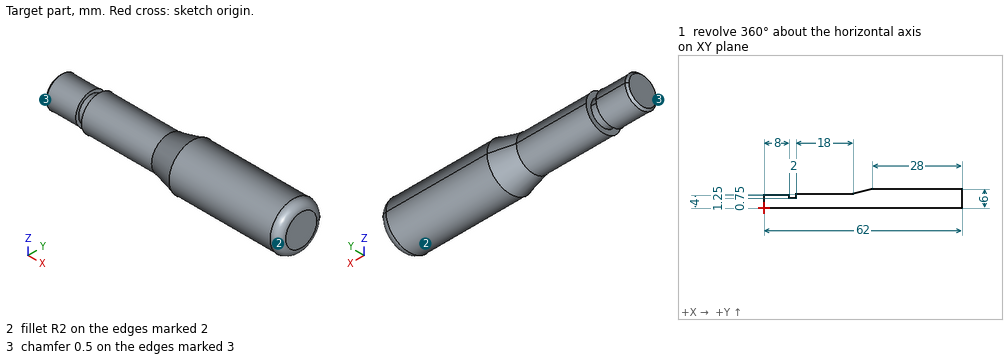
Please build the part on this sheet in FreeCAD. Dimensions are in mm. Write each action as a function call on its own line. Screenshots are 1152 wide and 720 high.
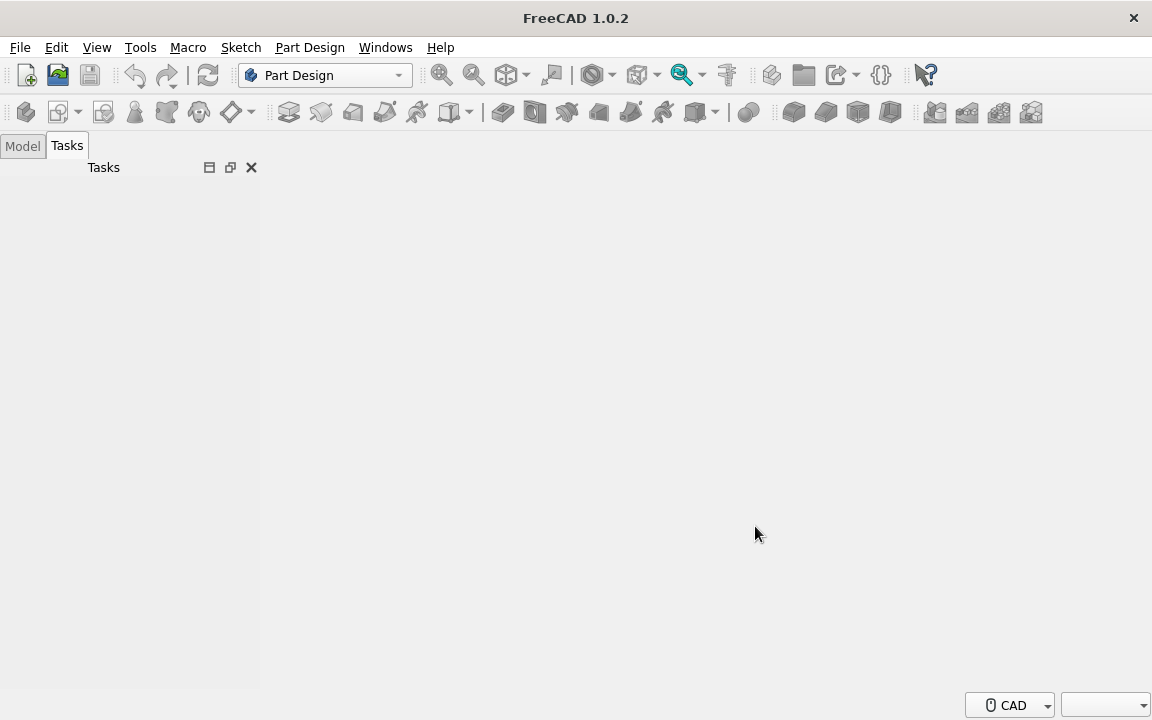
click(26, 76)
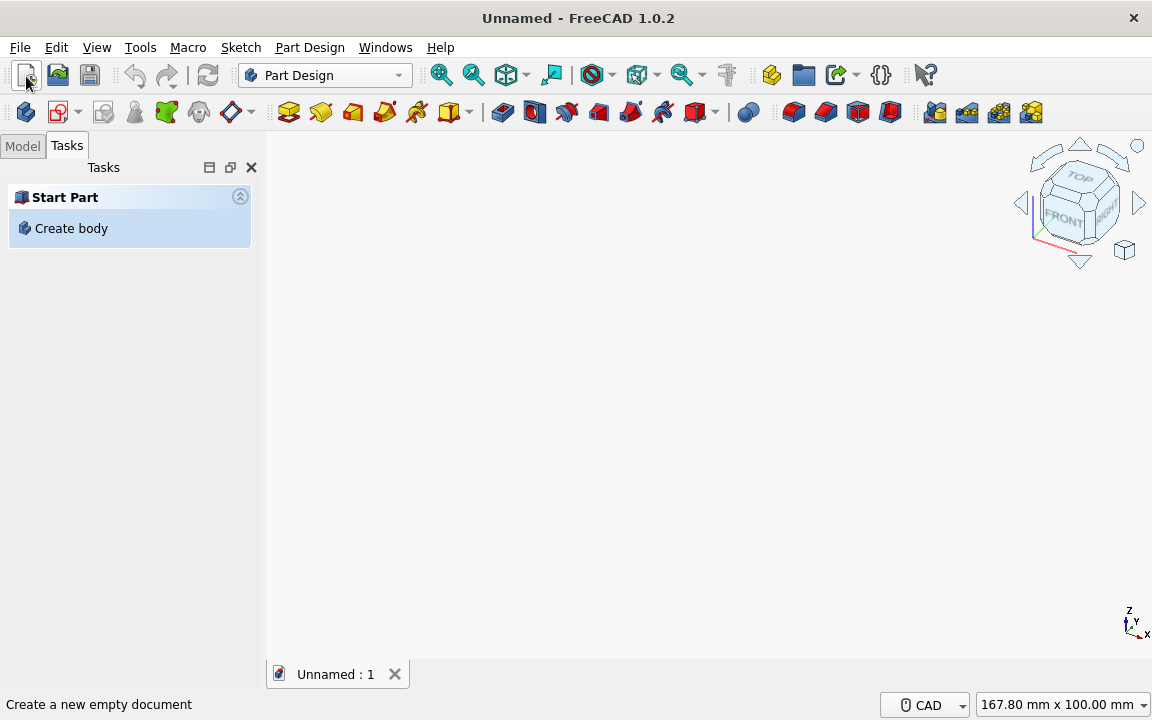
click(58, 112)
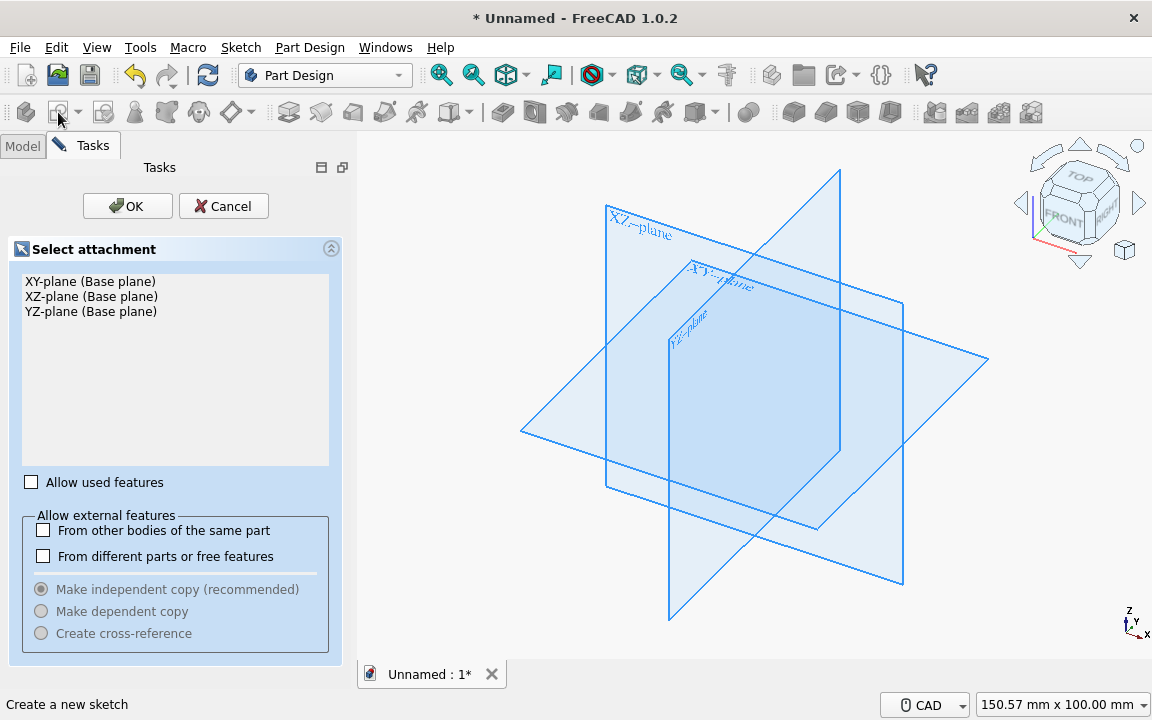
click(82, 282)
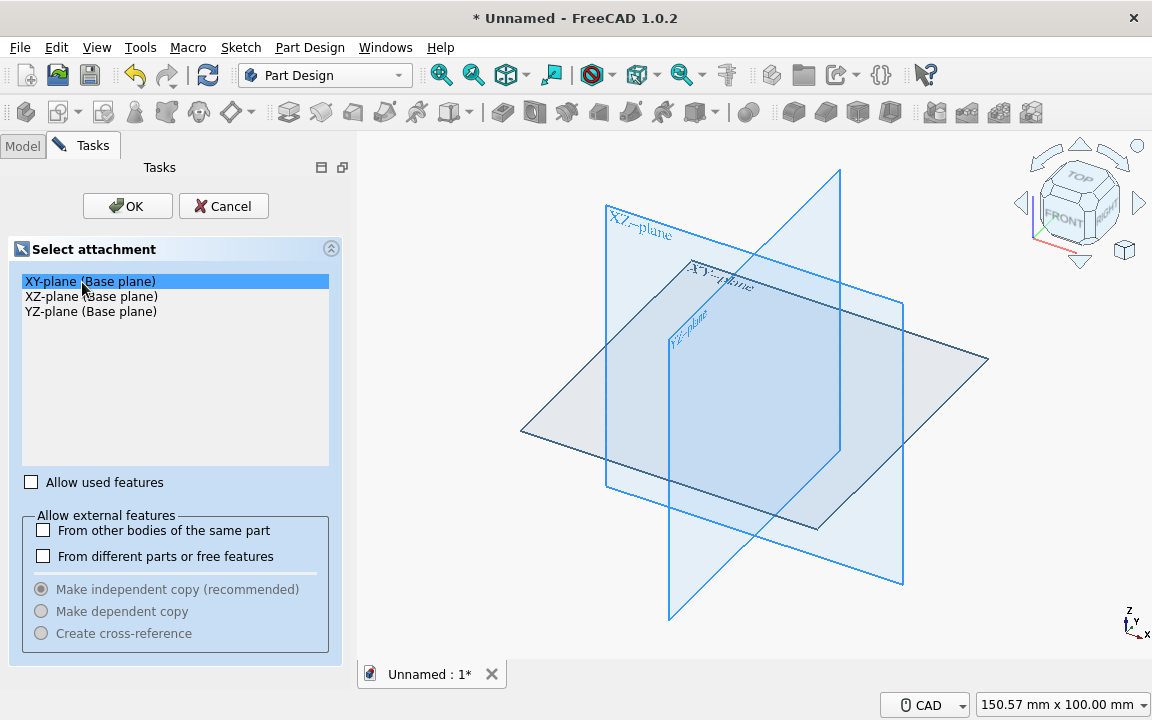
click(128, 206)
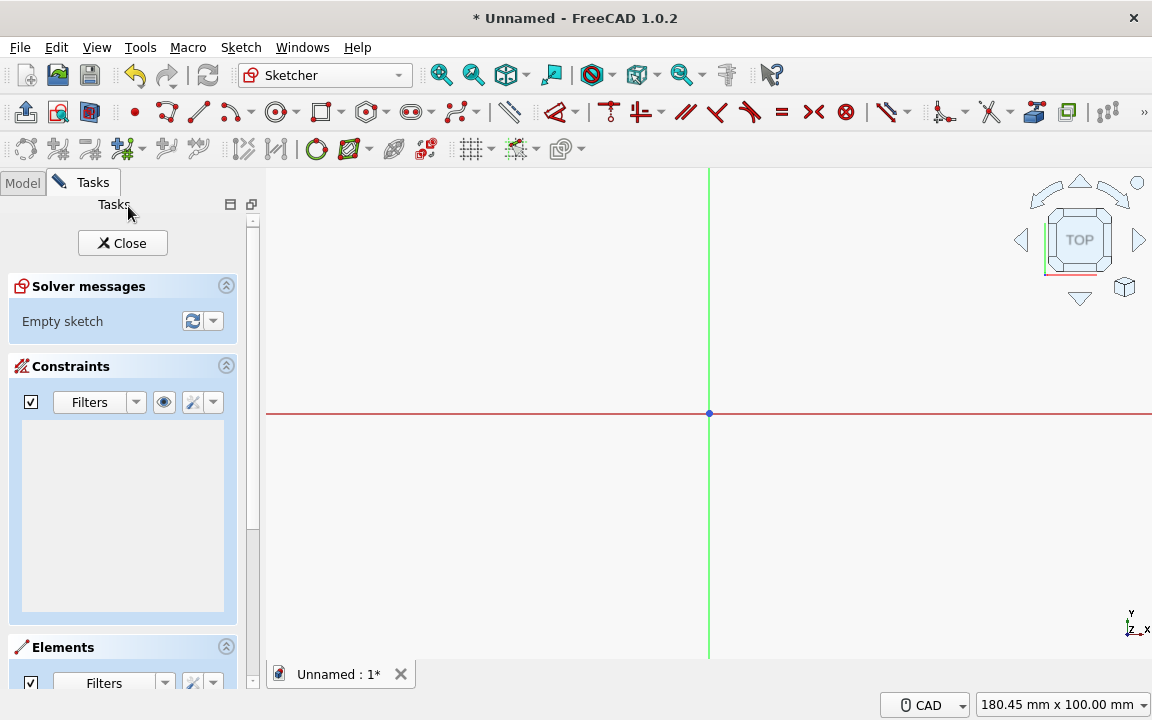
scroll(294, 480, down, 1)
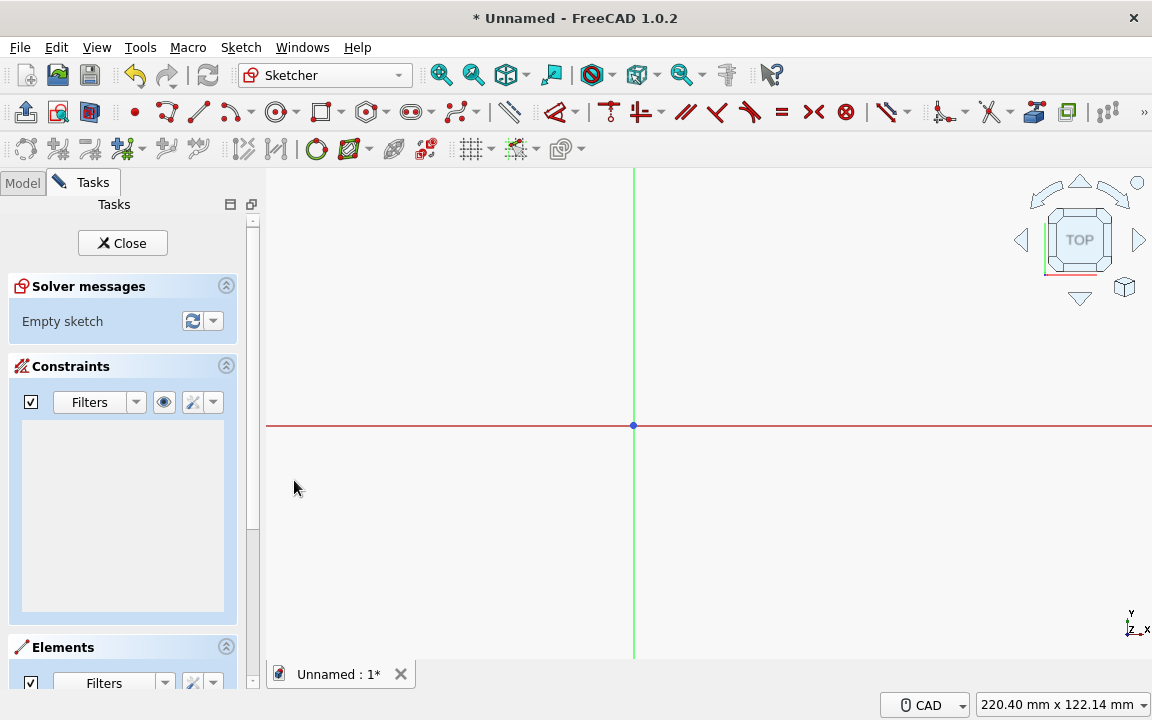
scroll(902, 414, up, 3)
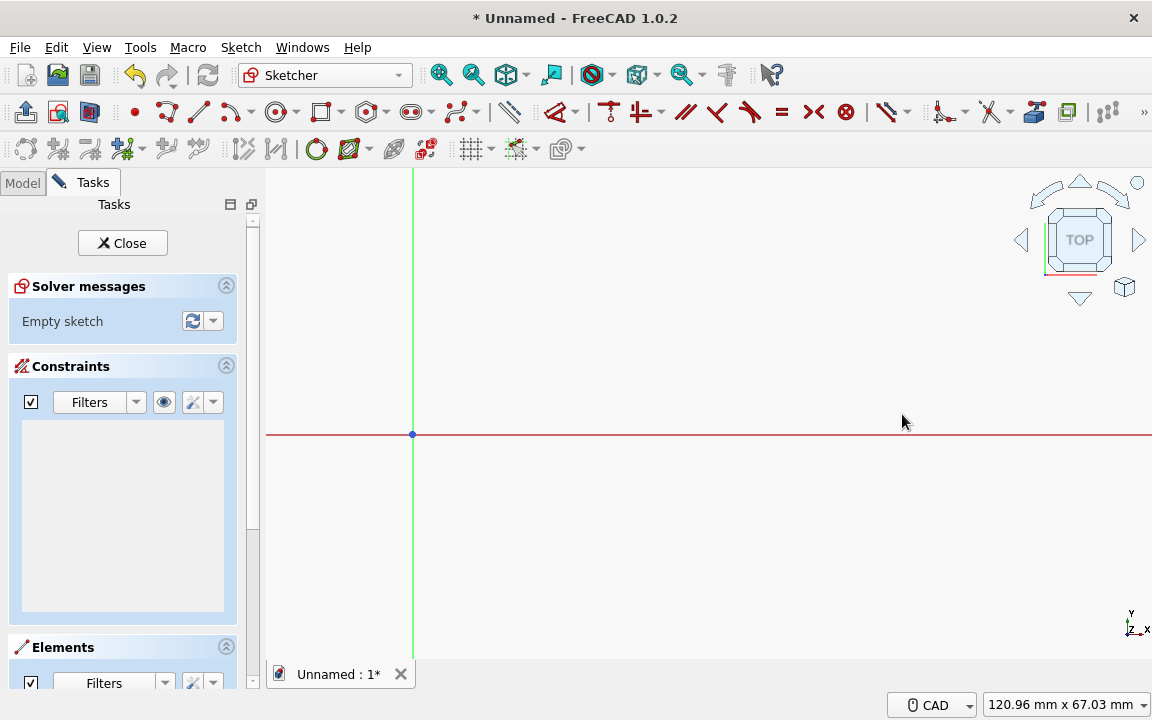
click(168, 112)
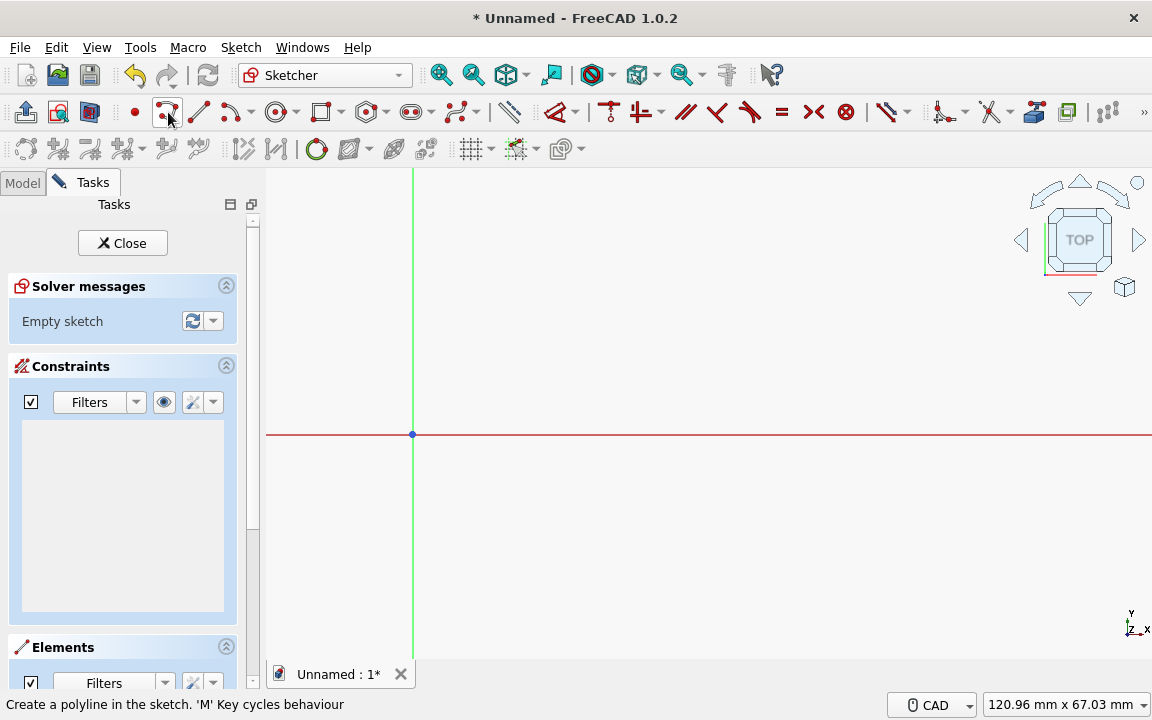
click(413, 435)
click(867, 426)
click(867, 391)
click(662, 391)
click(618, 402)
click(486, 402)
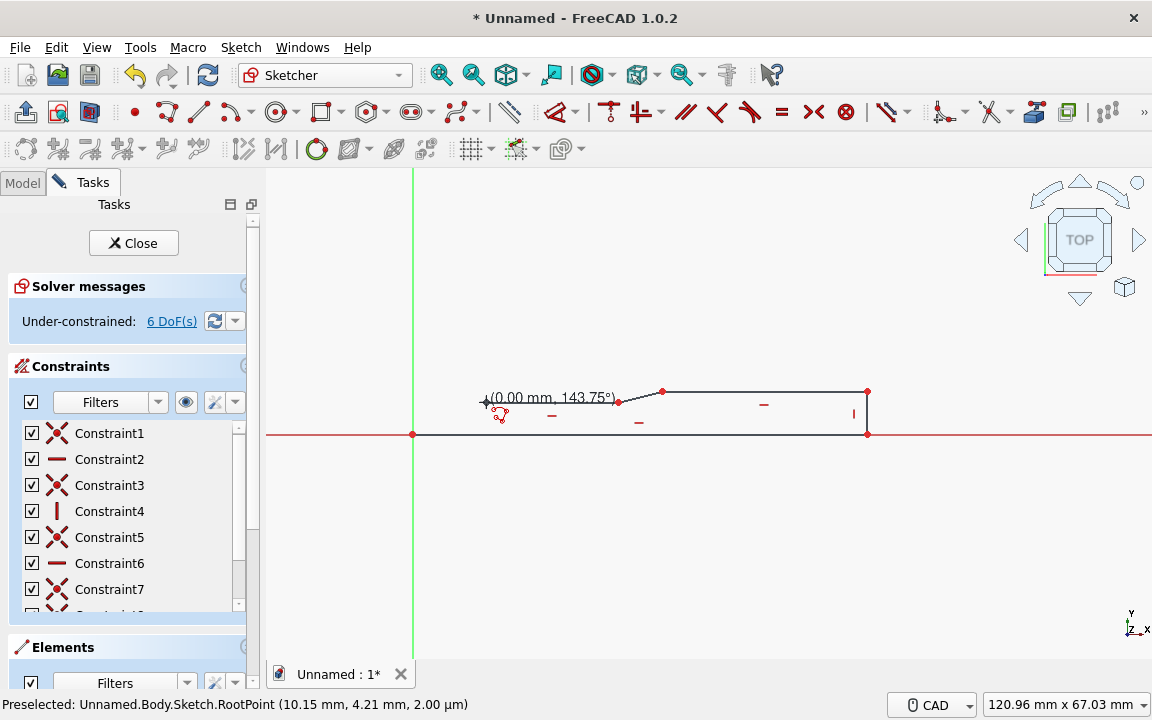
scroll(486, 411, up, 3)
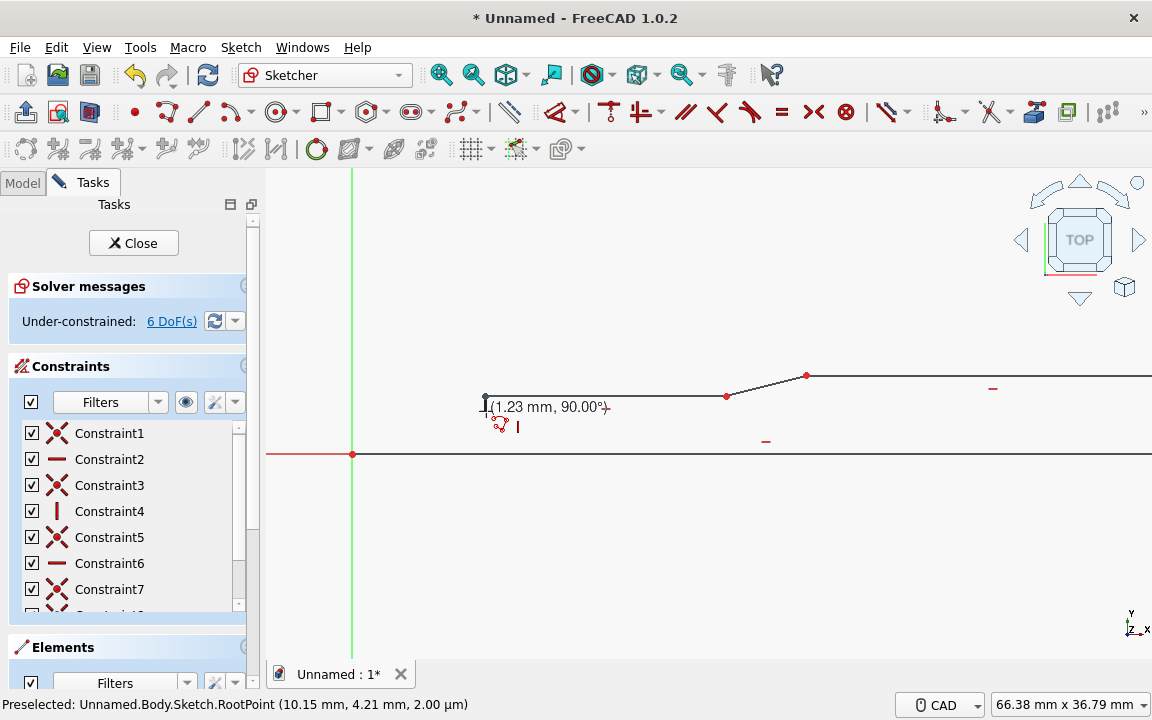
click(486, 411)
click(459, 411)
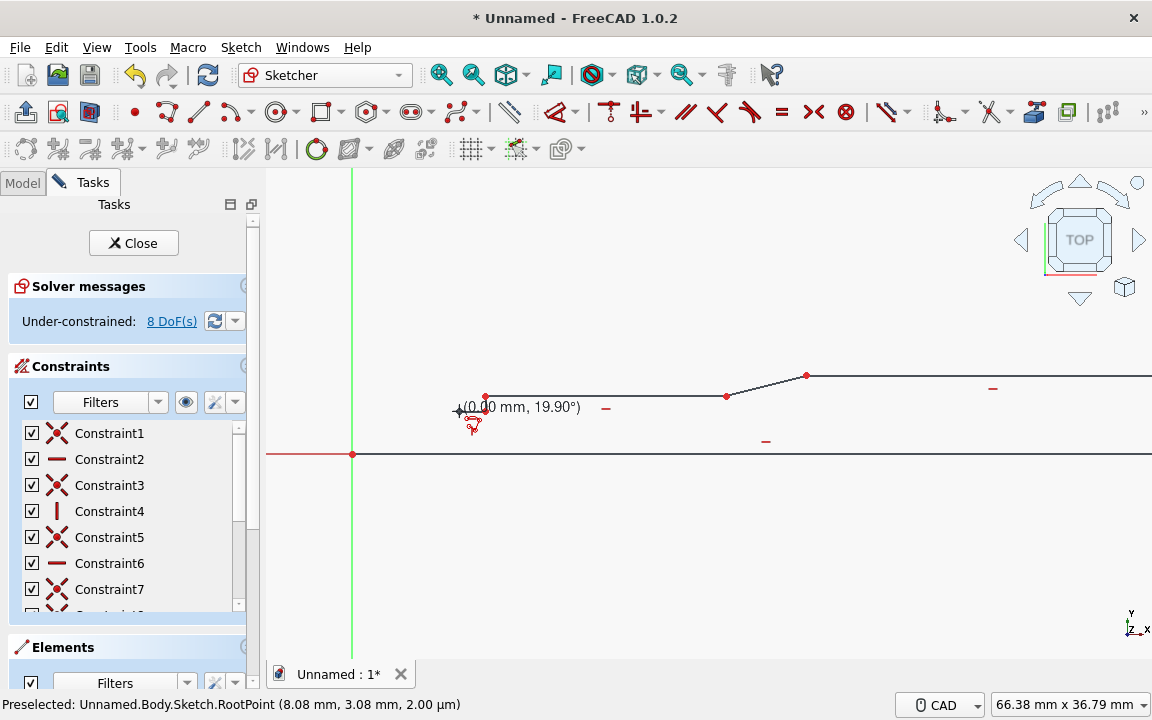
scroll(459, 401, up, 3)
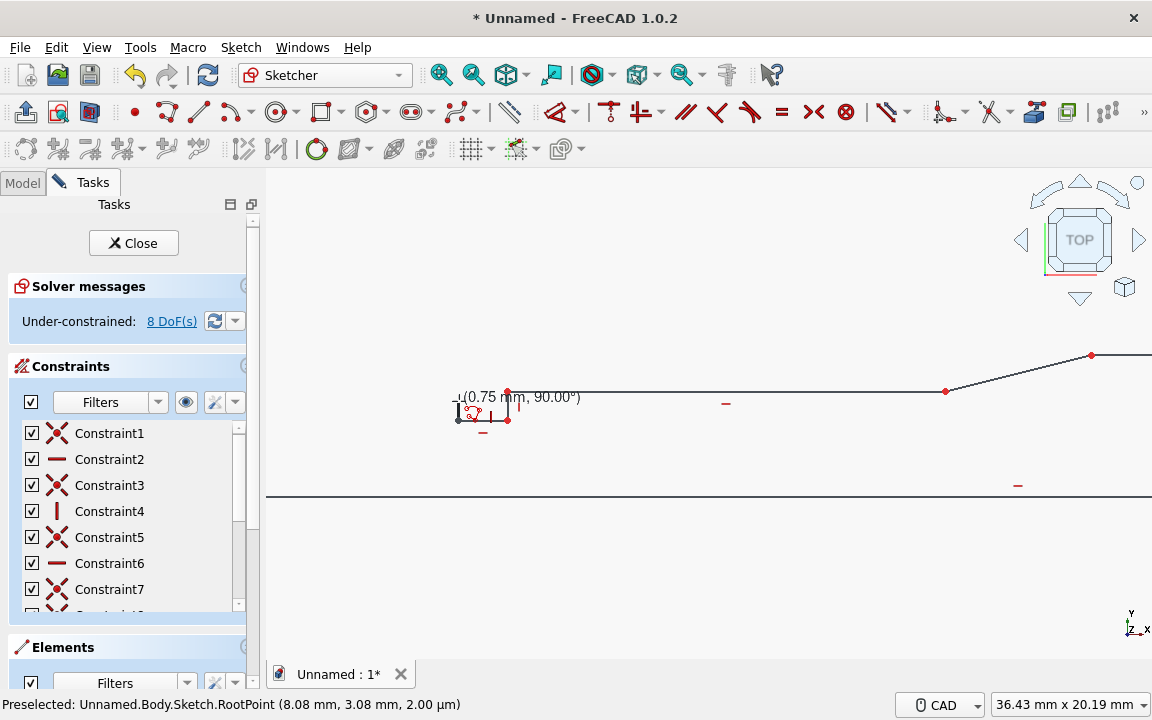
click(459, 400)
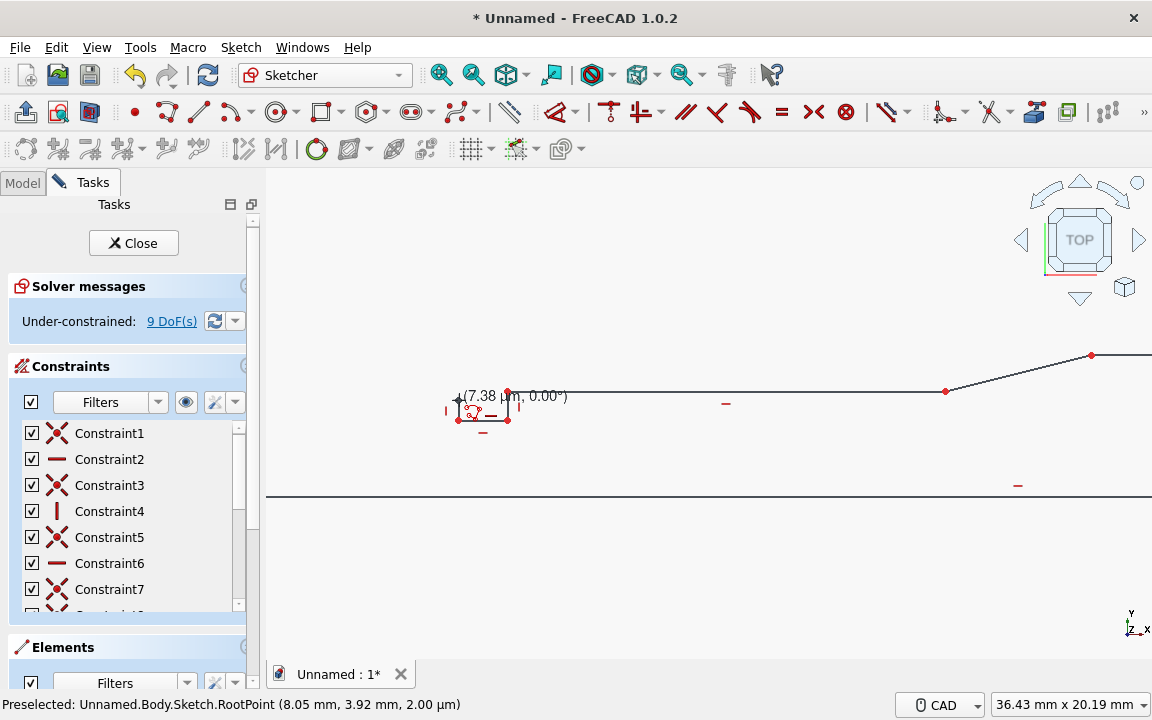
scroll(478, 409, down, 6)